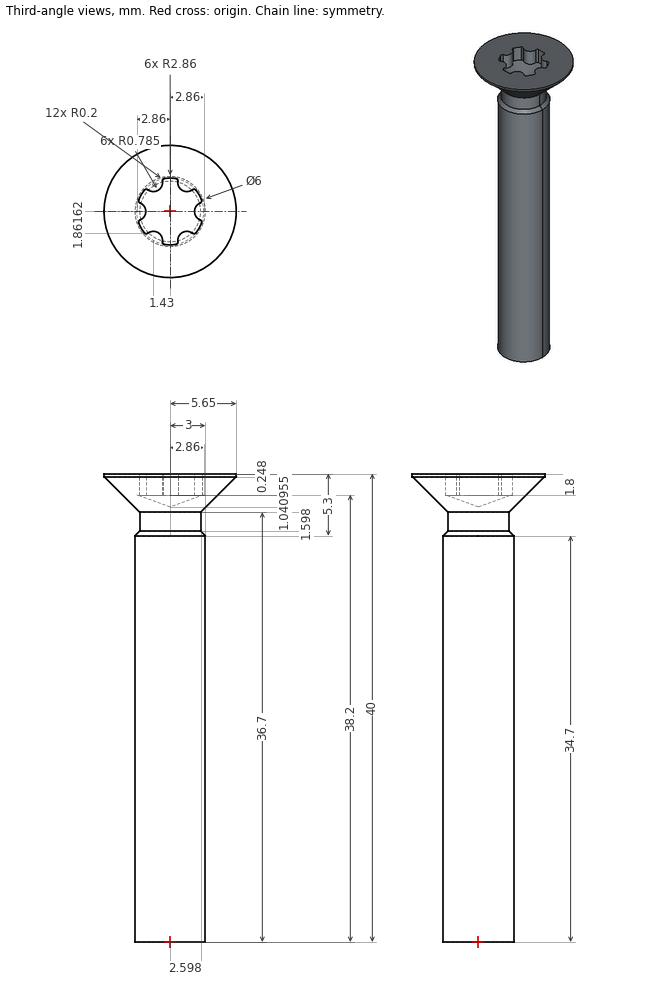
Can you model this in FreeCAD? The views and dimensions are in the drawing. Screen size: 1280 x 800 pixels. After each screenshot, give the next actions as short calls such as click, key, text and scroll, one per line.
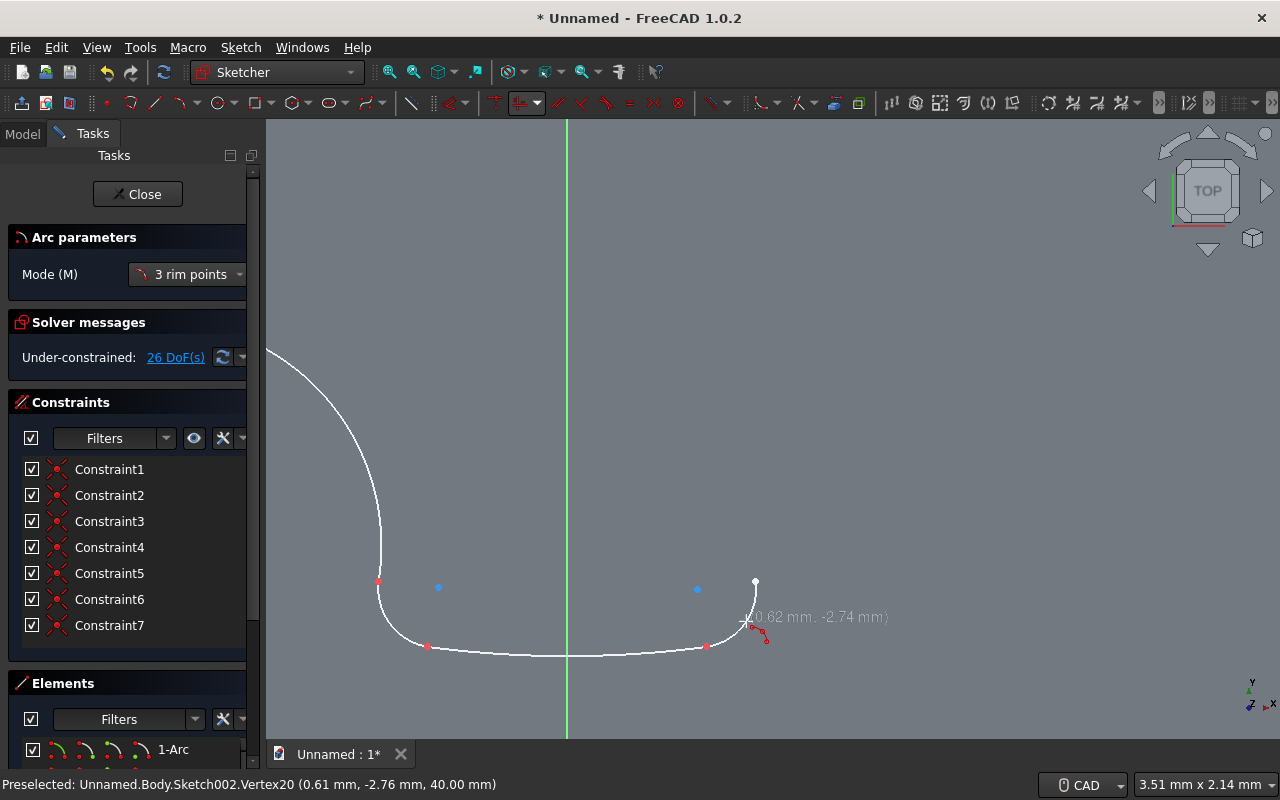
scroll(749, 625, down, 7)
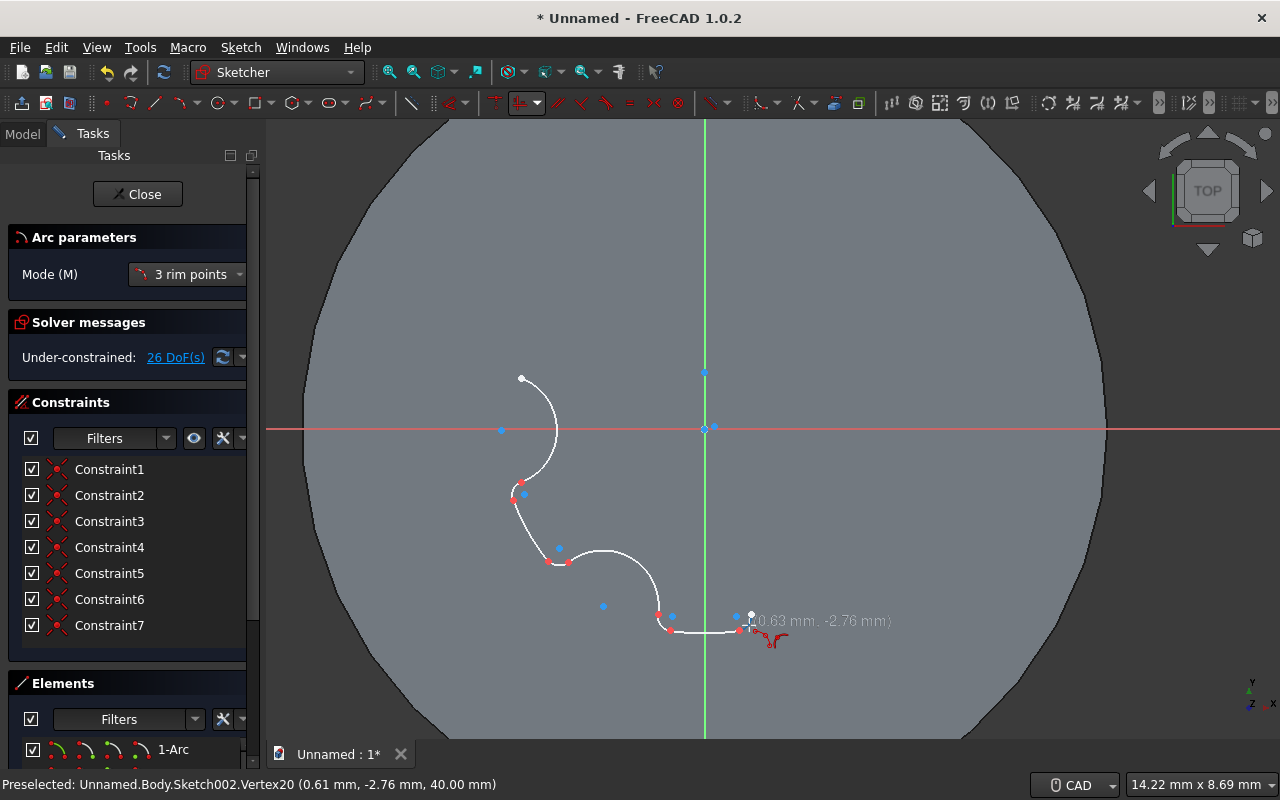
click(751, 615)
click(841, 562)
click(779, 557)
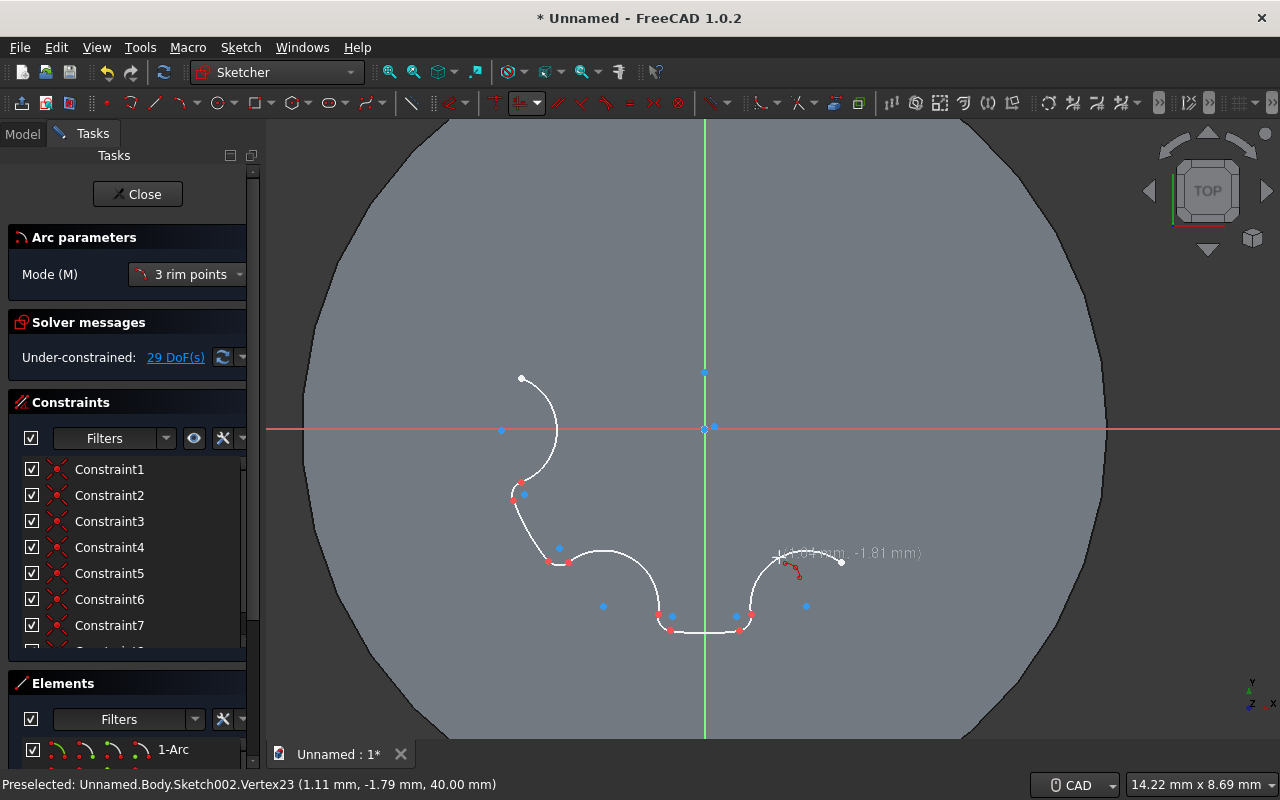
click(841, 563)
click(861, 560)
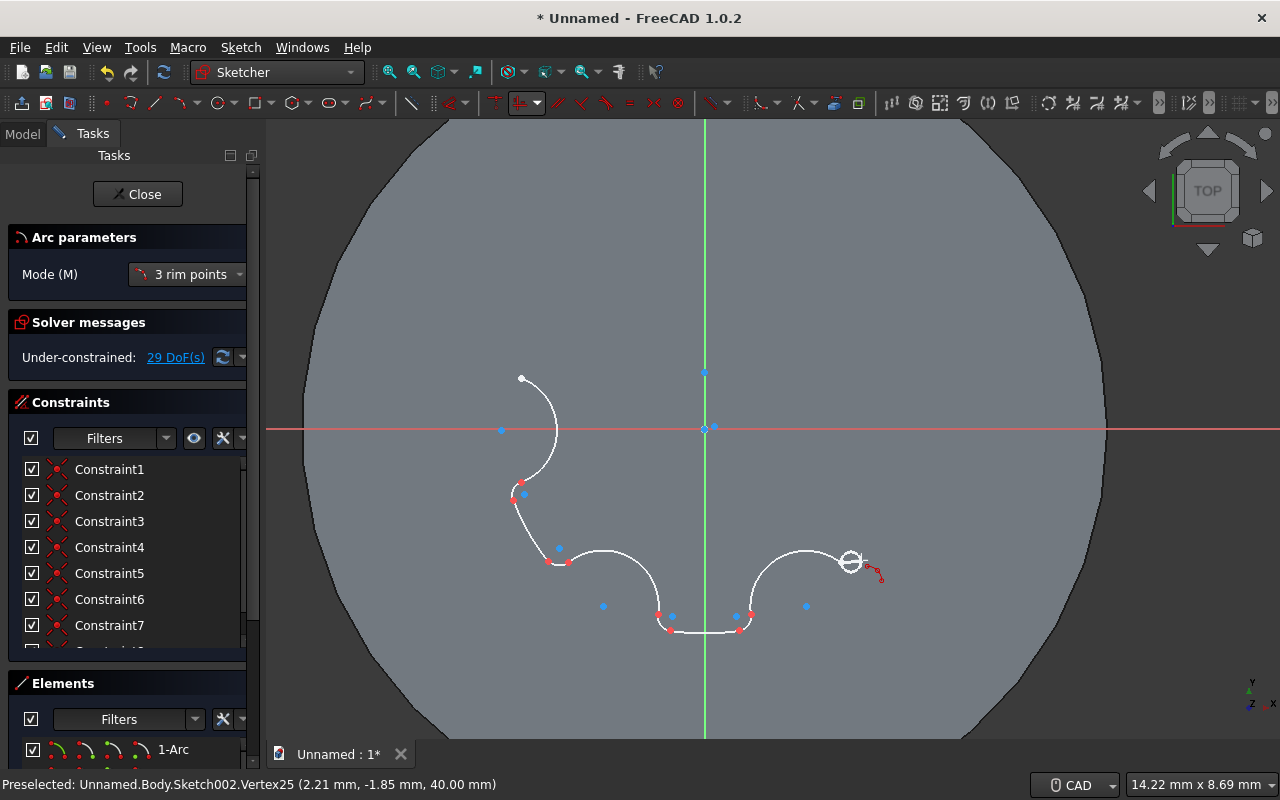
scroll(852, 565, up, 7)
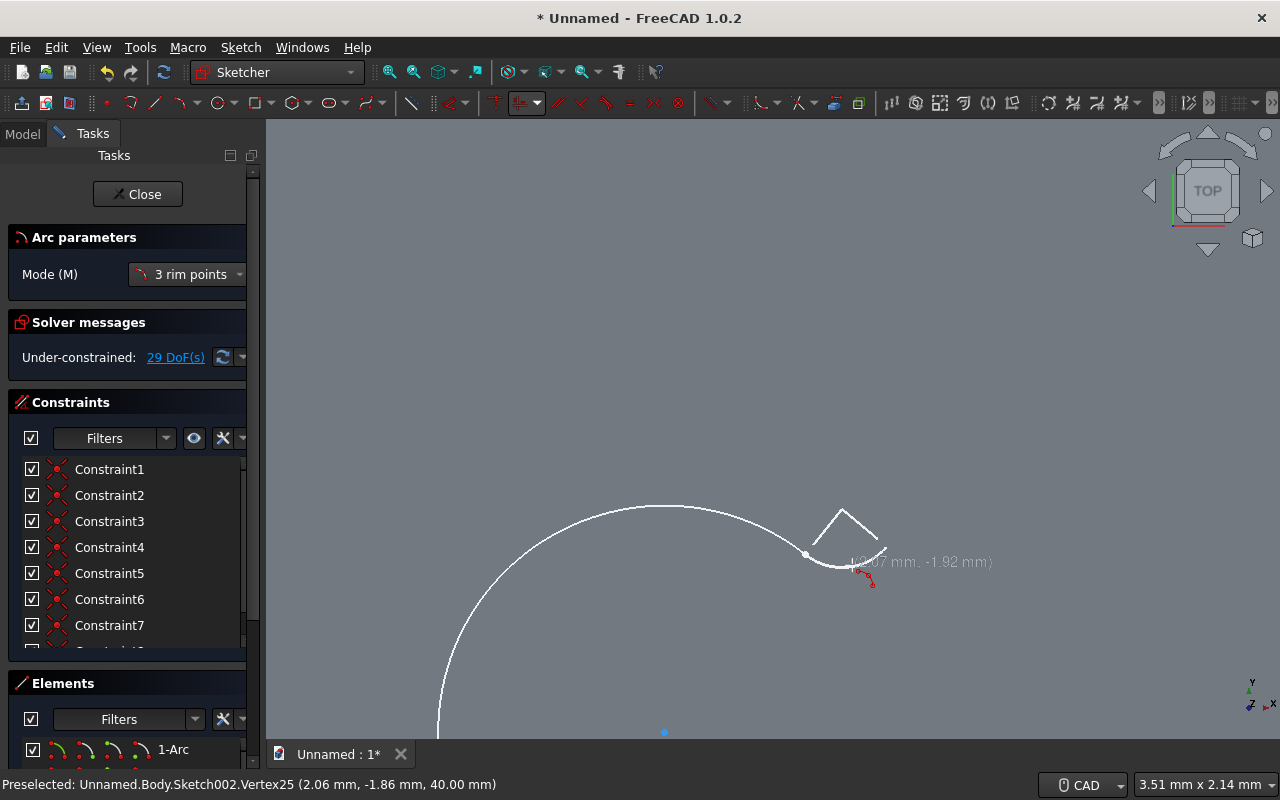
click(849, 563)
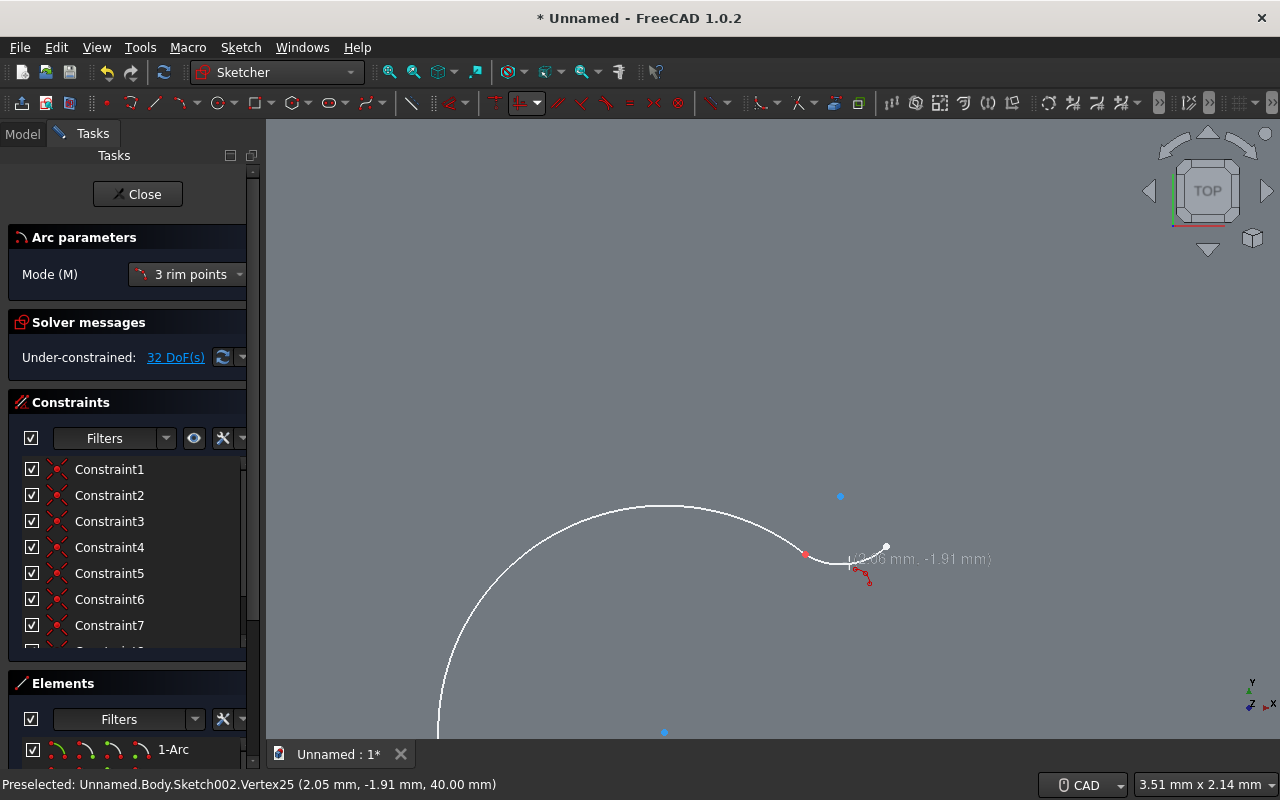
scroll(853, 565, down, 7)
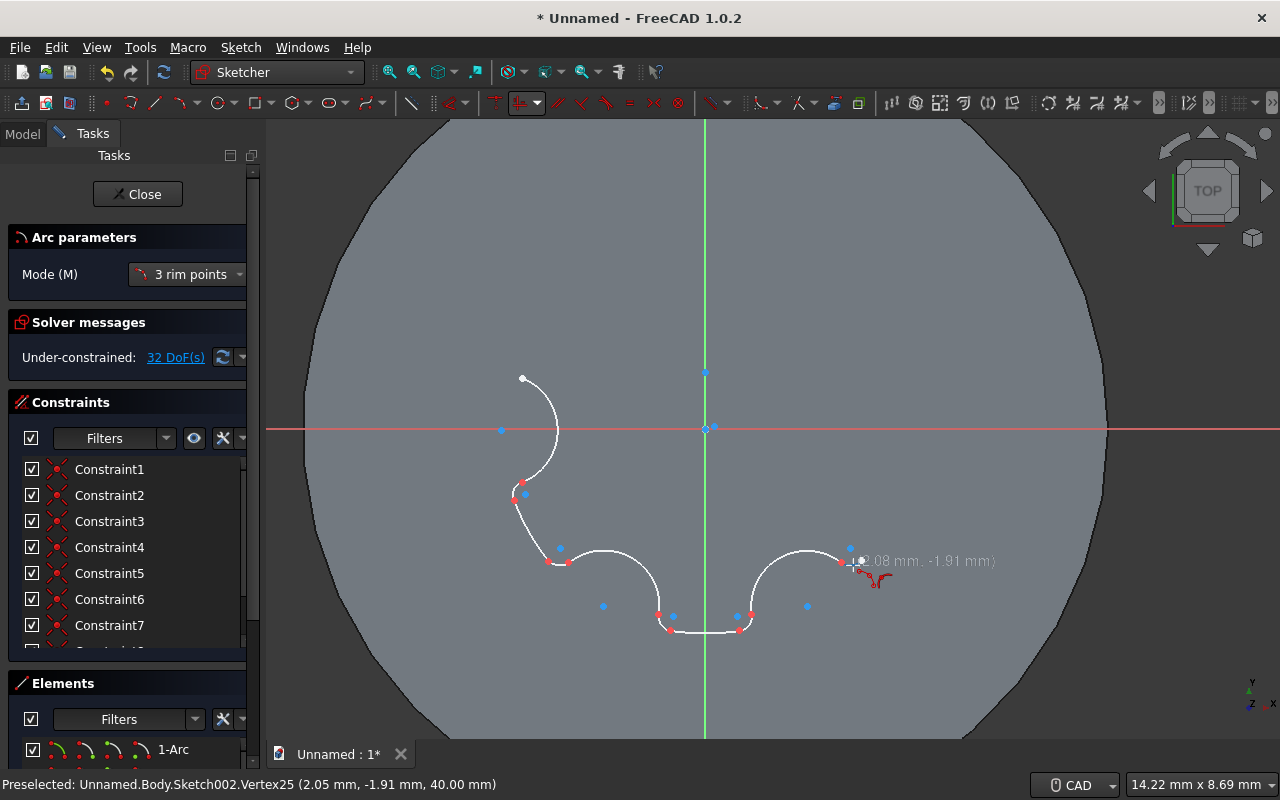
click(862, 561)
click(897, 499)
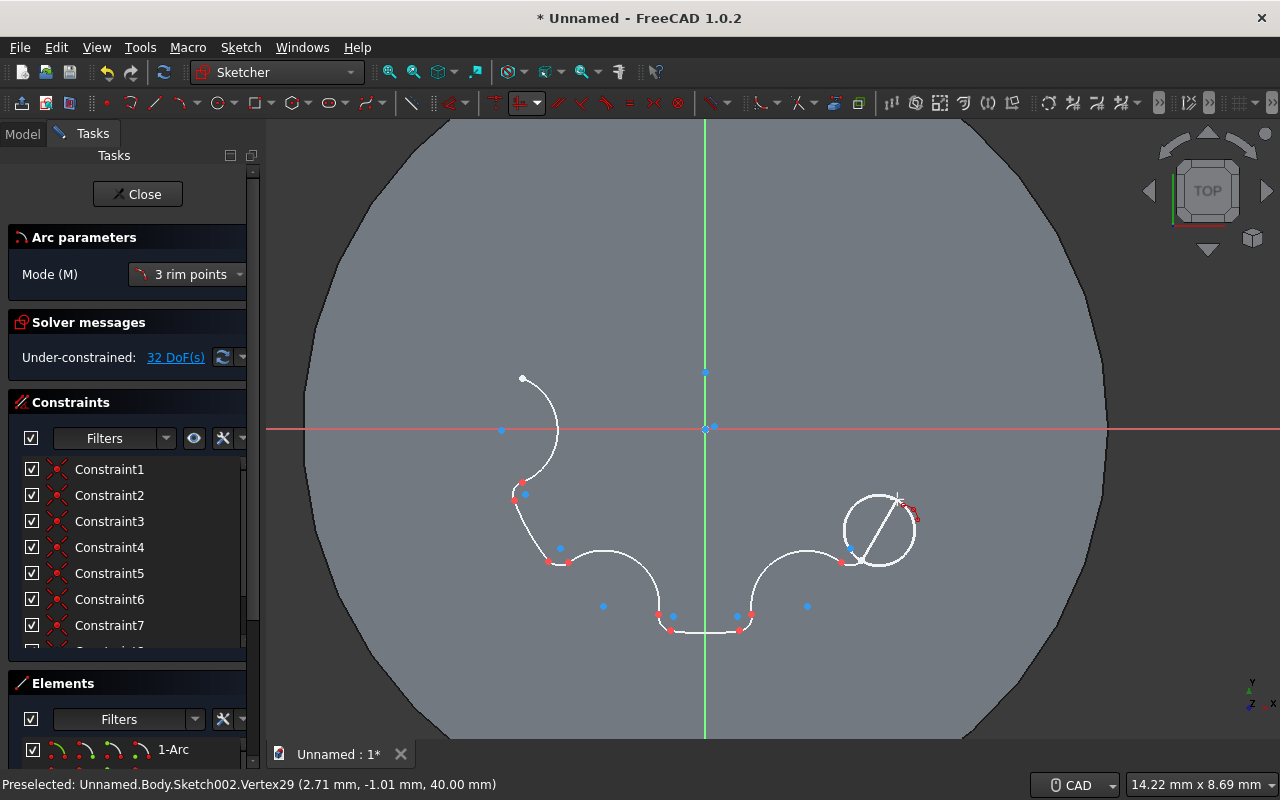
scroll(882, 531, up, 9)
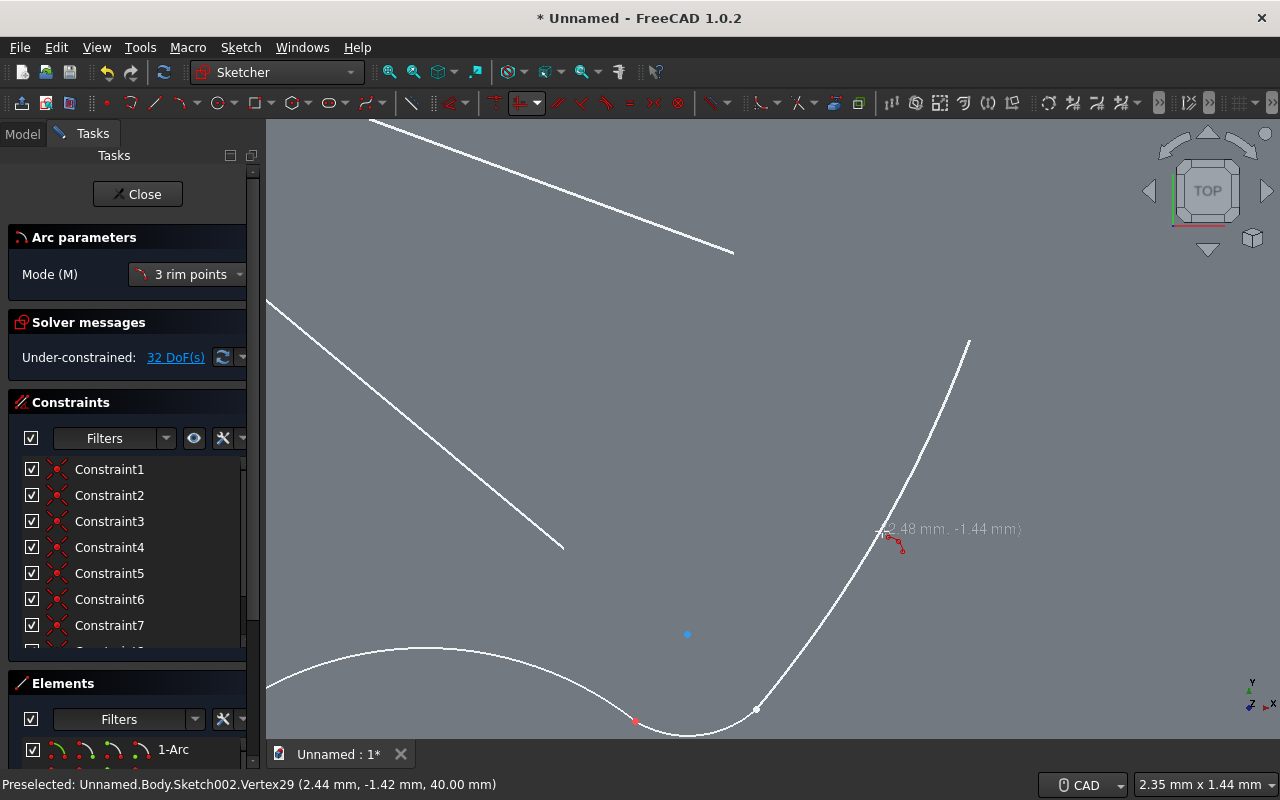
click(878, 529)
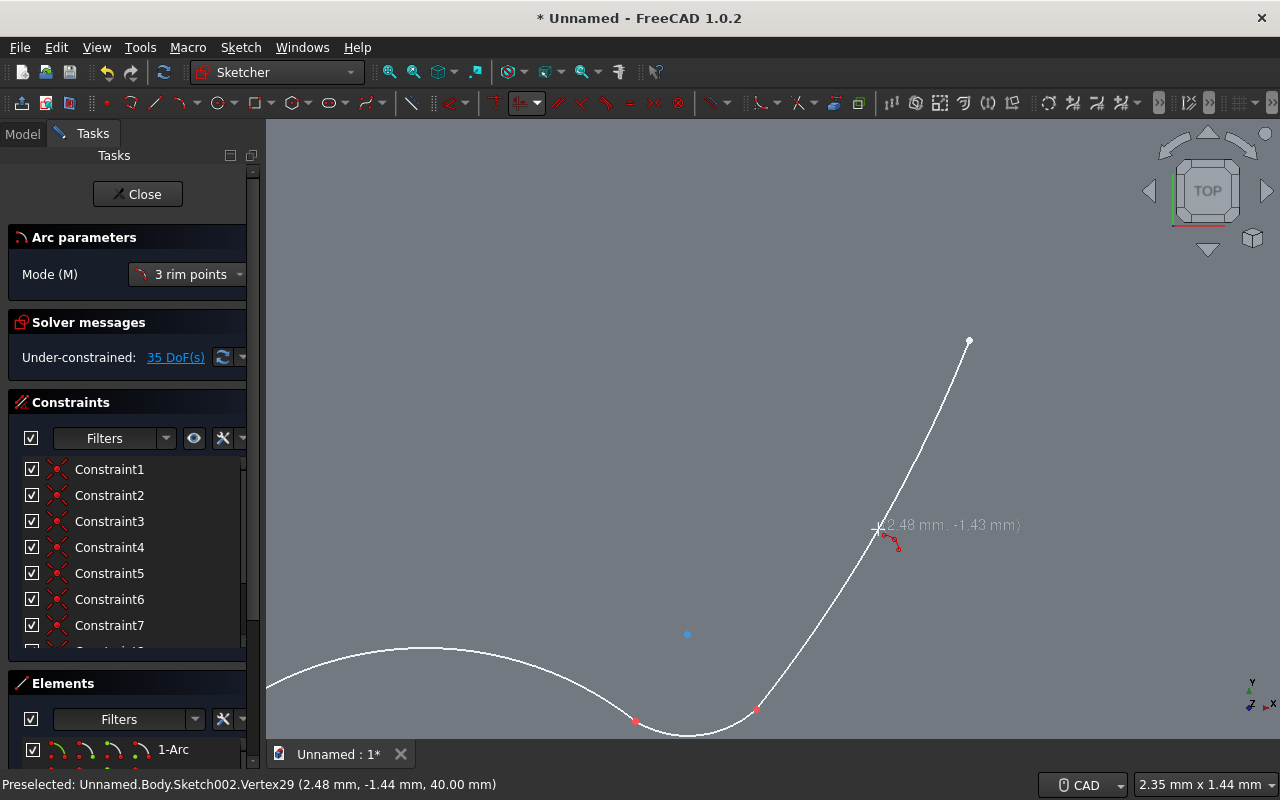
scroll(882, 531, down, 9)